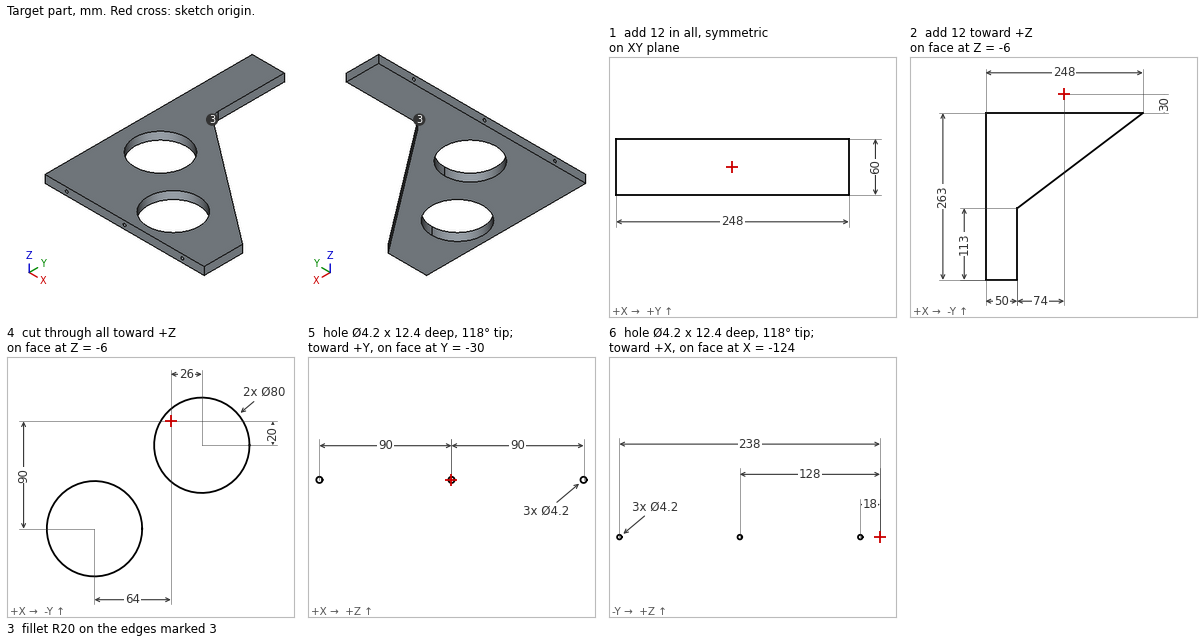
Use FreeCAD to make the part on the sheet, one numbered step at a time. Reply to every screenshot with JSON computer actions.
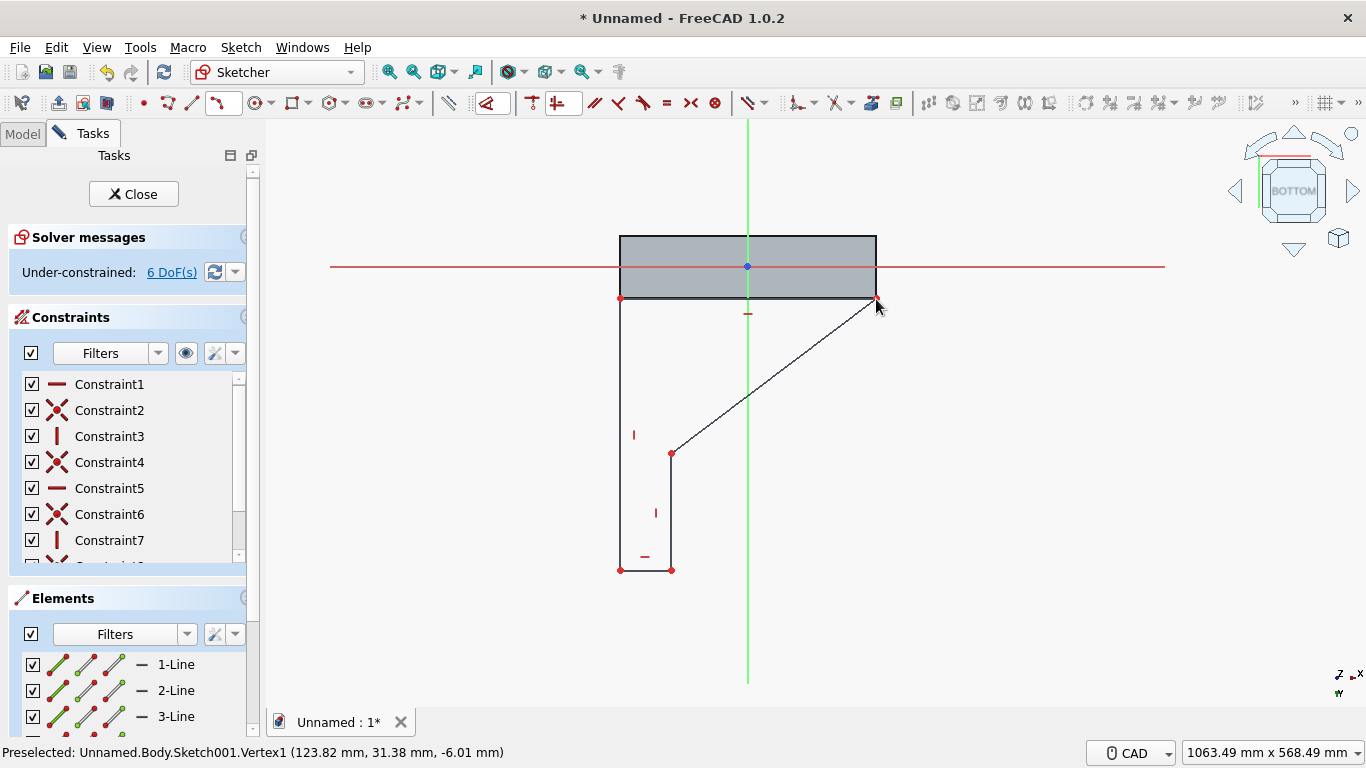
{"action": "left_click", "coordinate": [635, 571]}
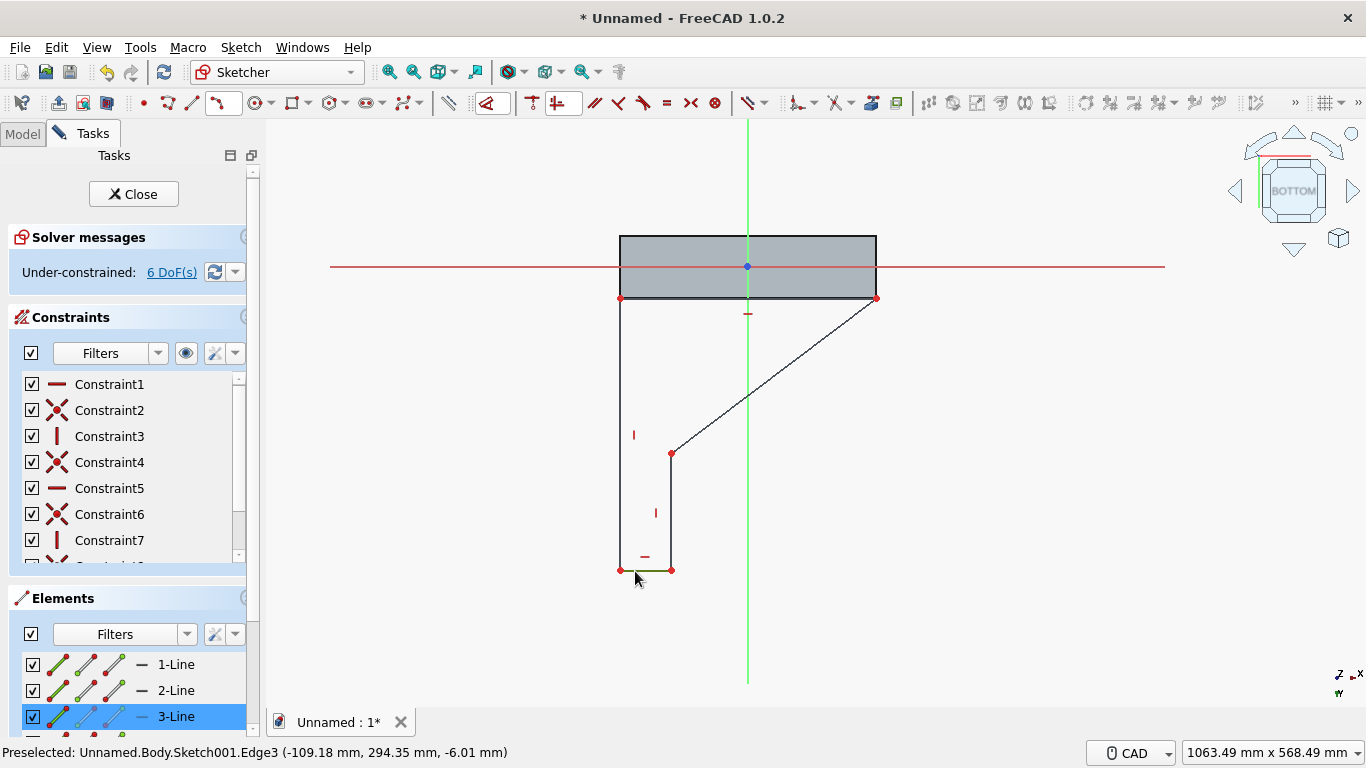
{"action": "left_click", "coordinate": [504, 104]}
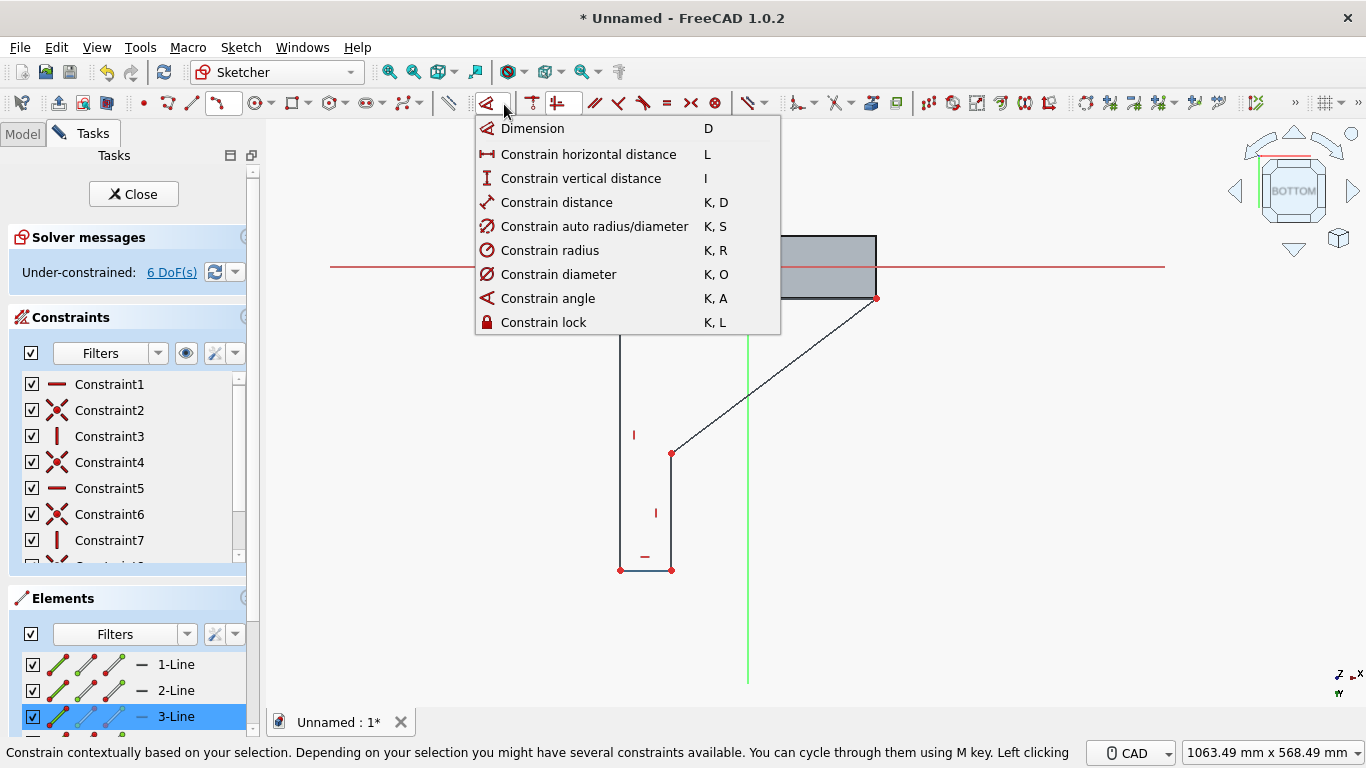
{"action": "left_click", "coordinate": [628, 154]}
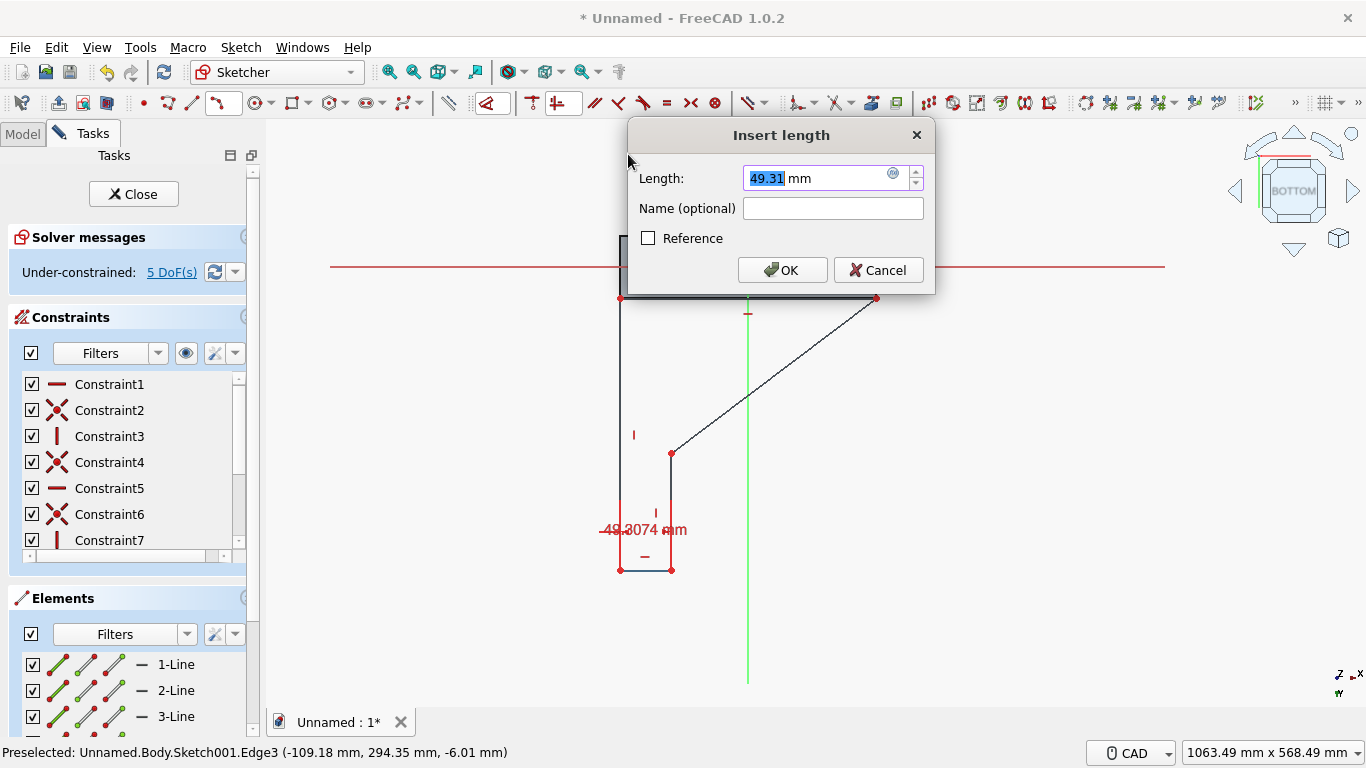
{"action": "type", "text": "50"}
{"action": "key", "text": "Return"}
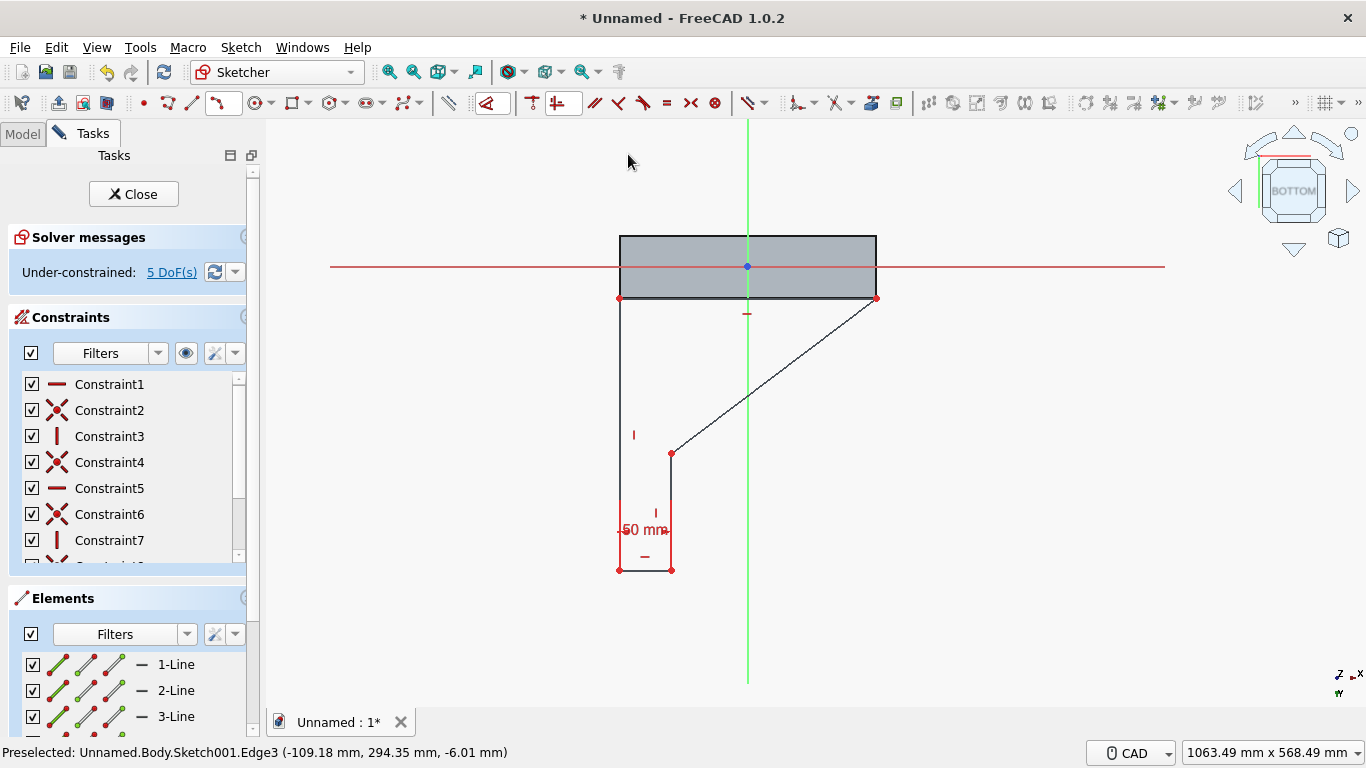
{"action": "left_click", "coordinate": [799, 299]}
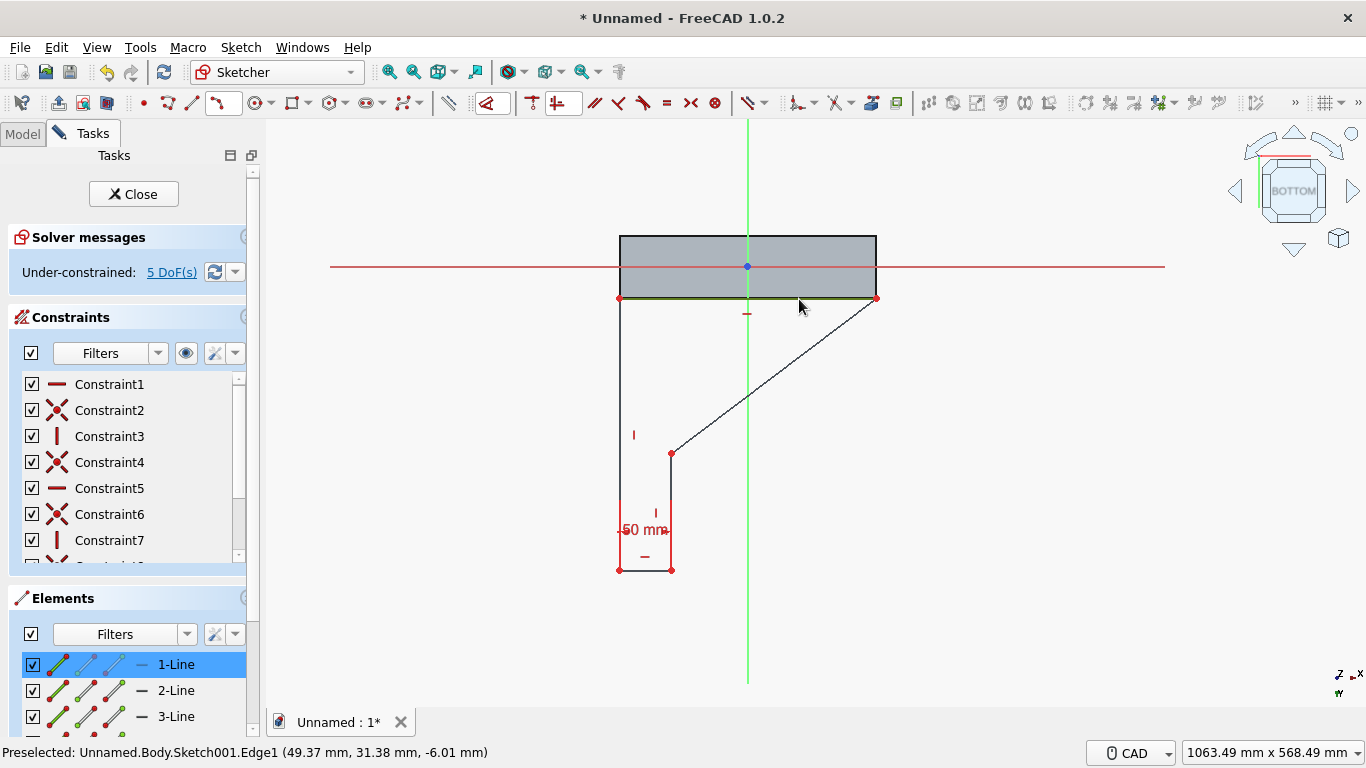
{"action": "key", "text": "l"}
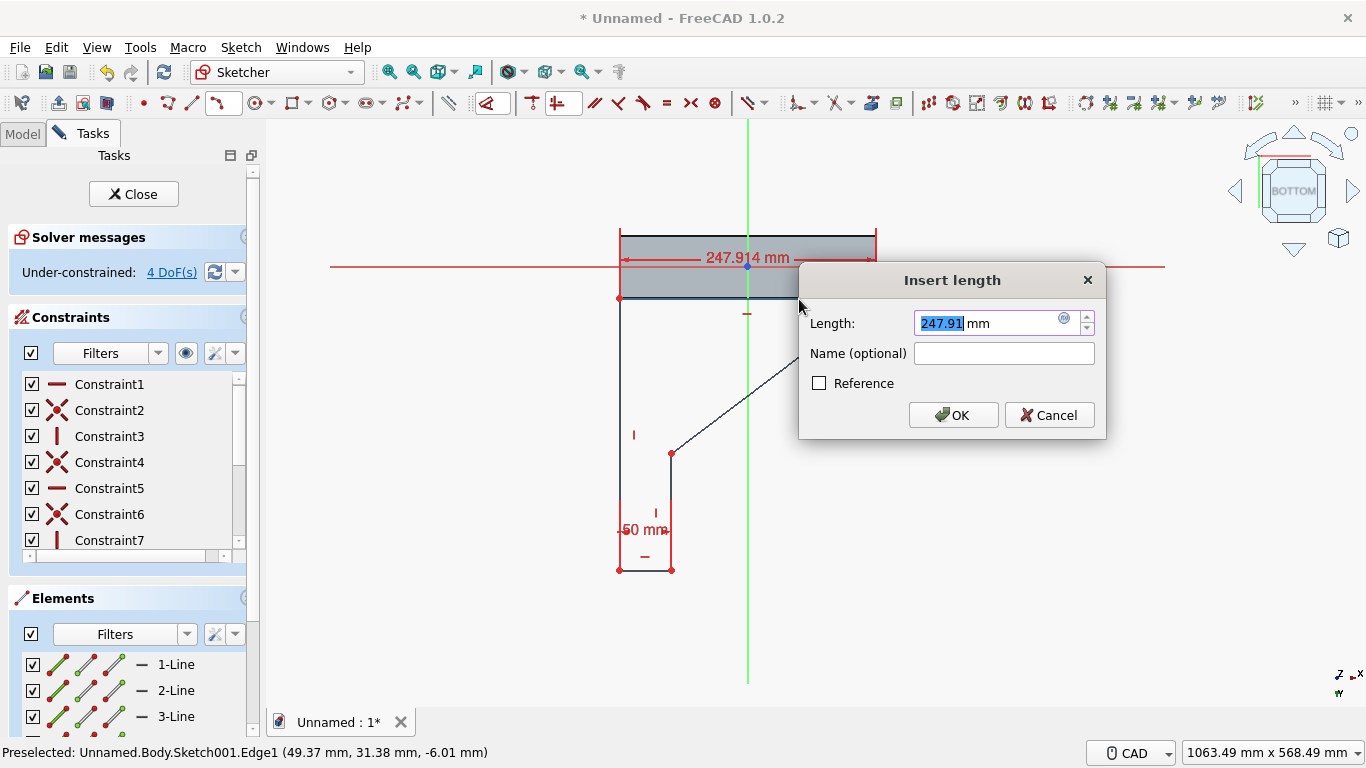
{"action": "type", "text": "248"}
{"action": "key", "text": "Return"}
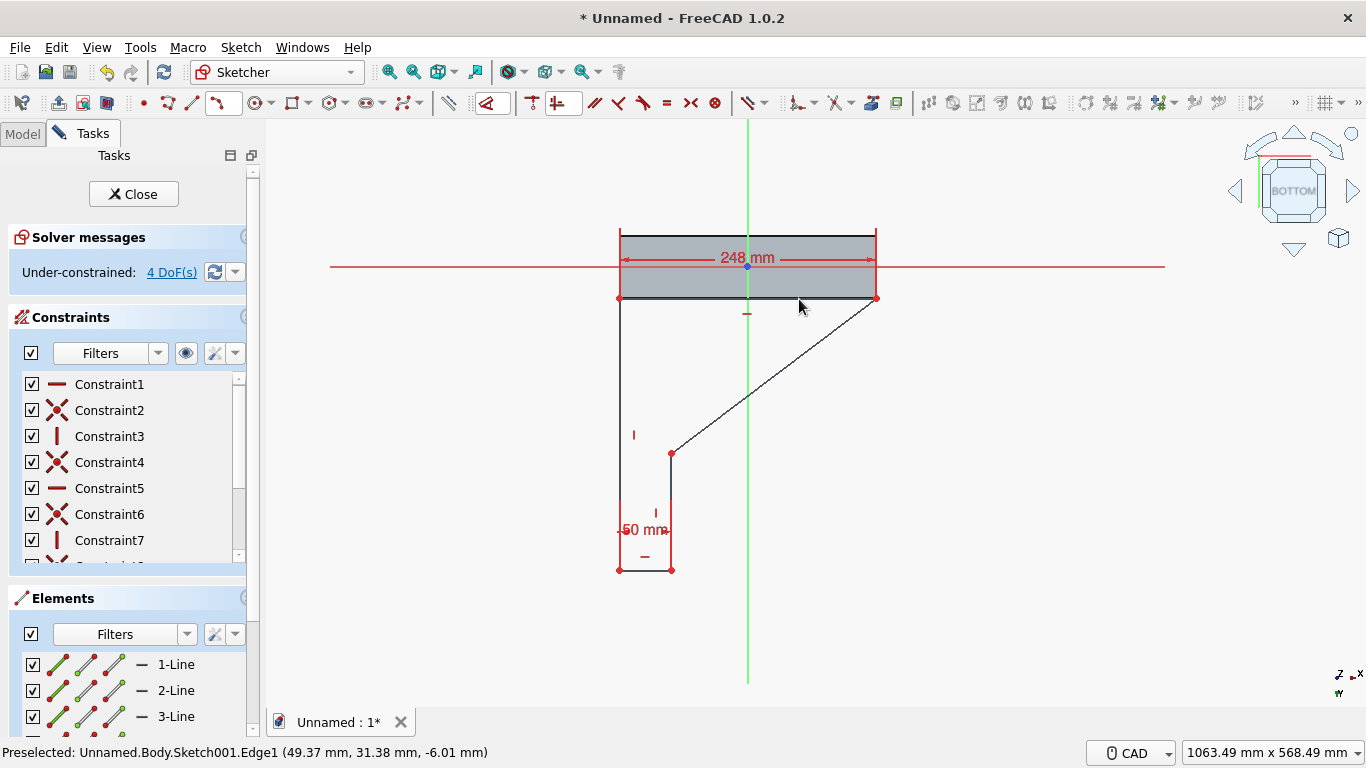
{"action": "left_click", "coordinate": [620, 381]}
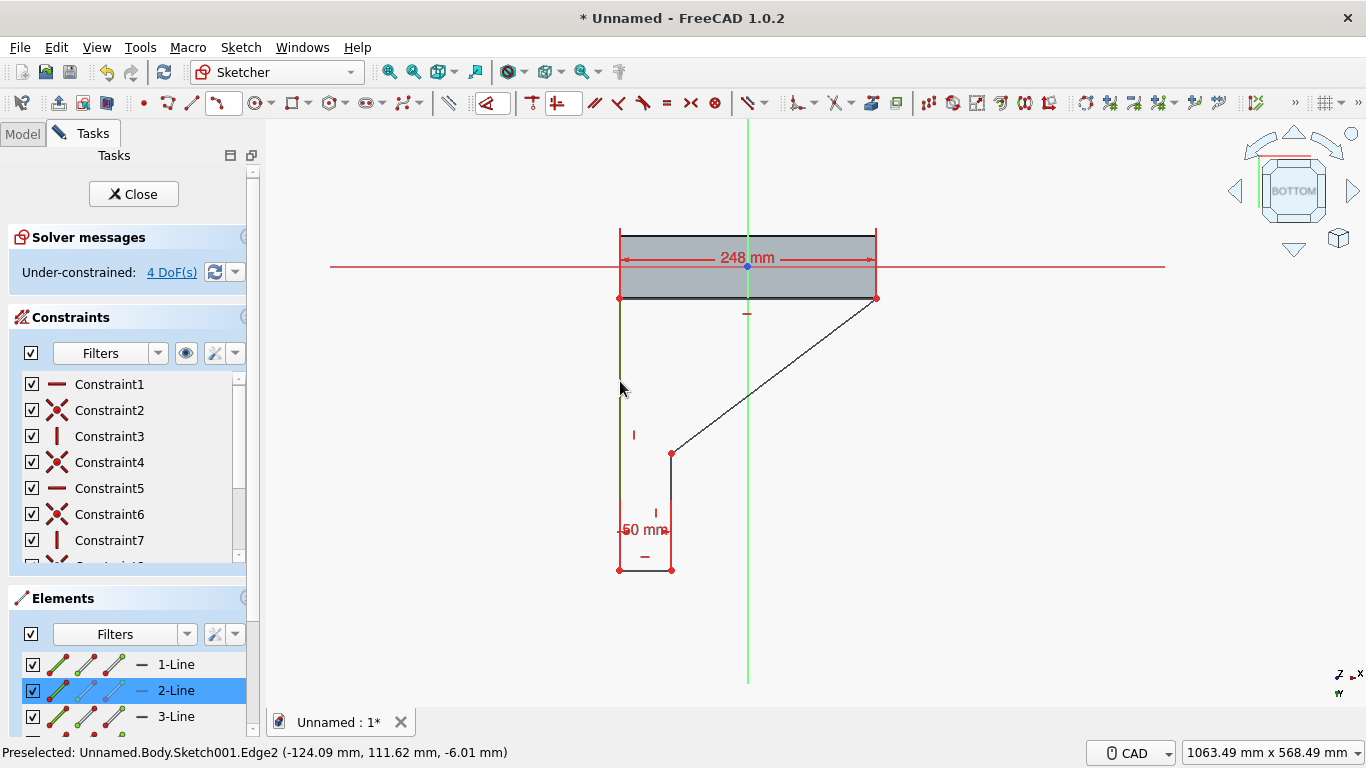
{"action": "left_click", "coordinate": [504, 104]}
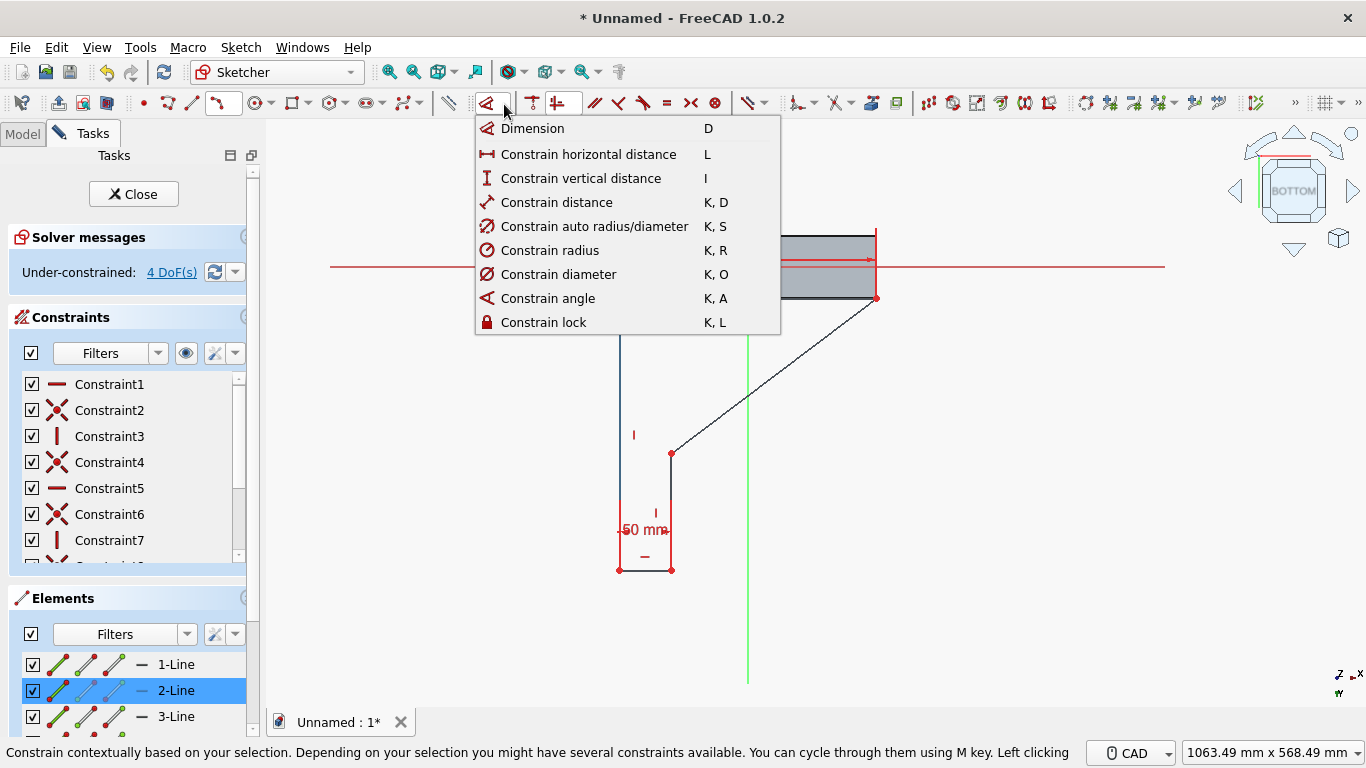
{"action": "left_click", "coordinate": [628, 178]}